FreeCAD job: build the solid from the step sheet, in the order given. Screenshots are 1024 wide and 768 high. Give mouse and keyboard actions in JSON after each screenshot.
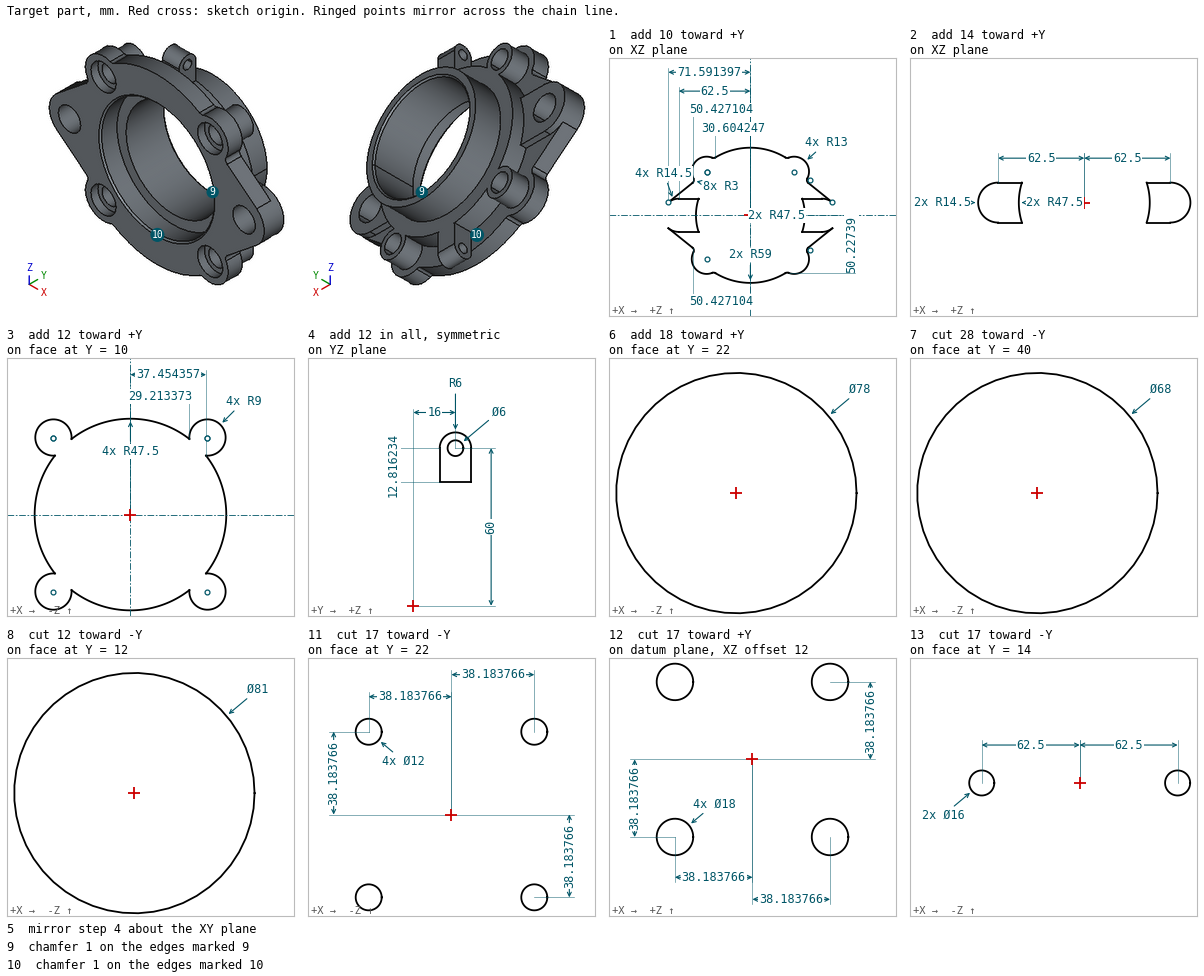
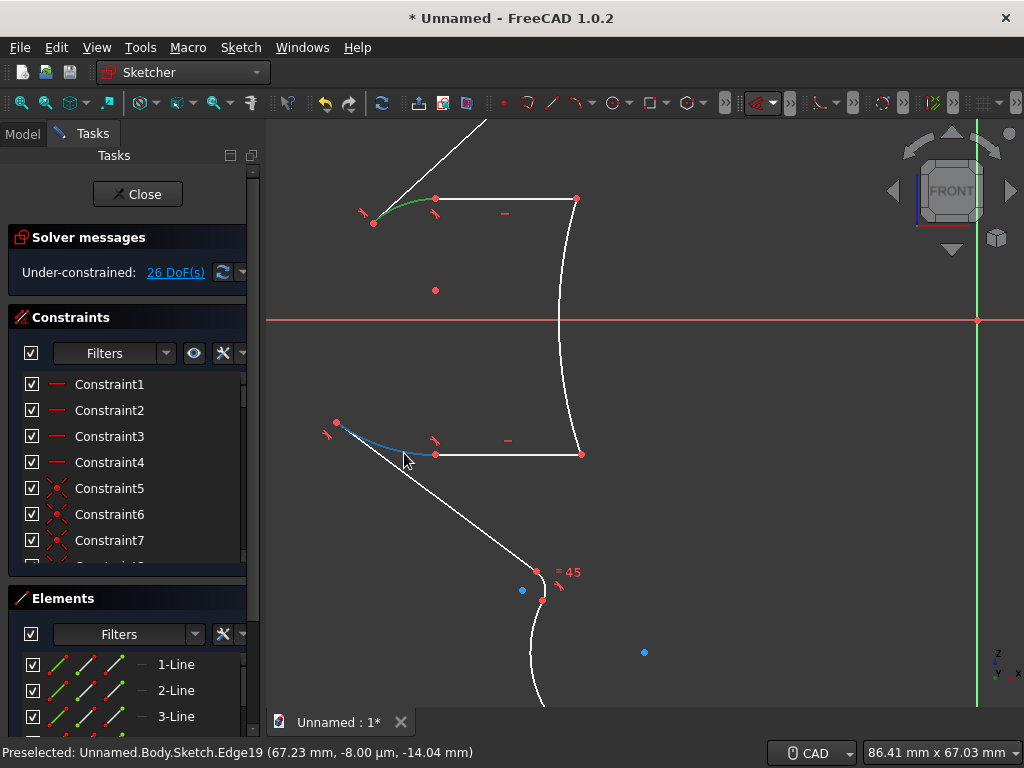
{"action": "left_click", "coordinate": [404, 452]}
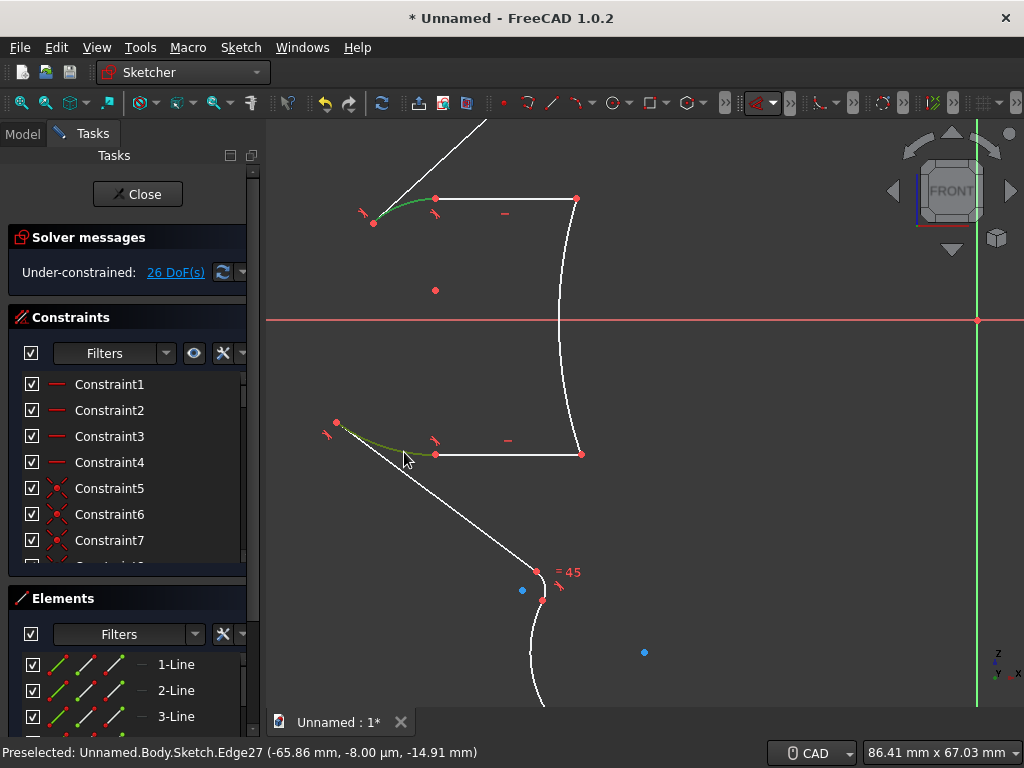
{"action": "key", "text": "e"}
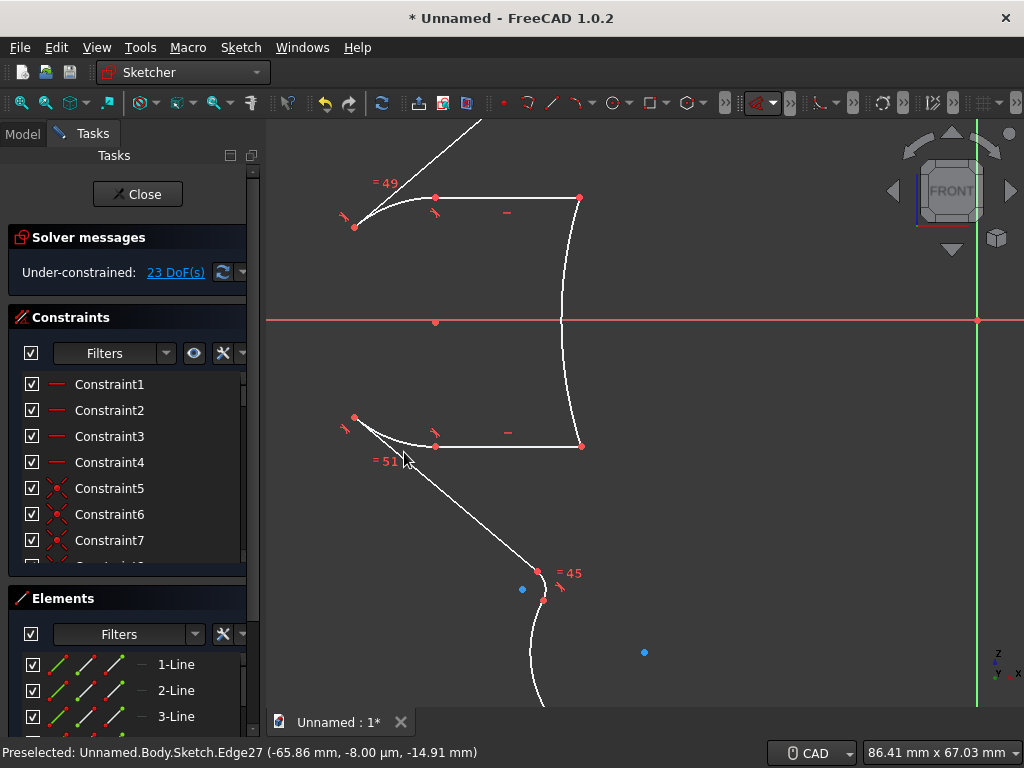
{"action": "scroll", "coordinate": [404, 453], "scroll_direction": "down", "scroll_amount": 6}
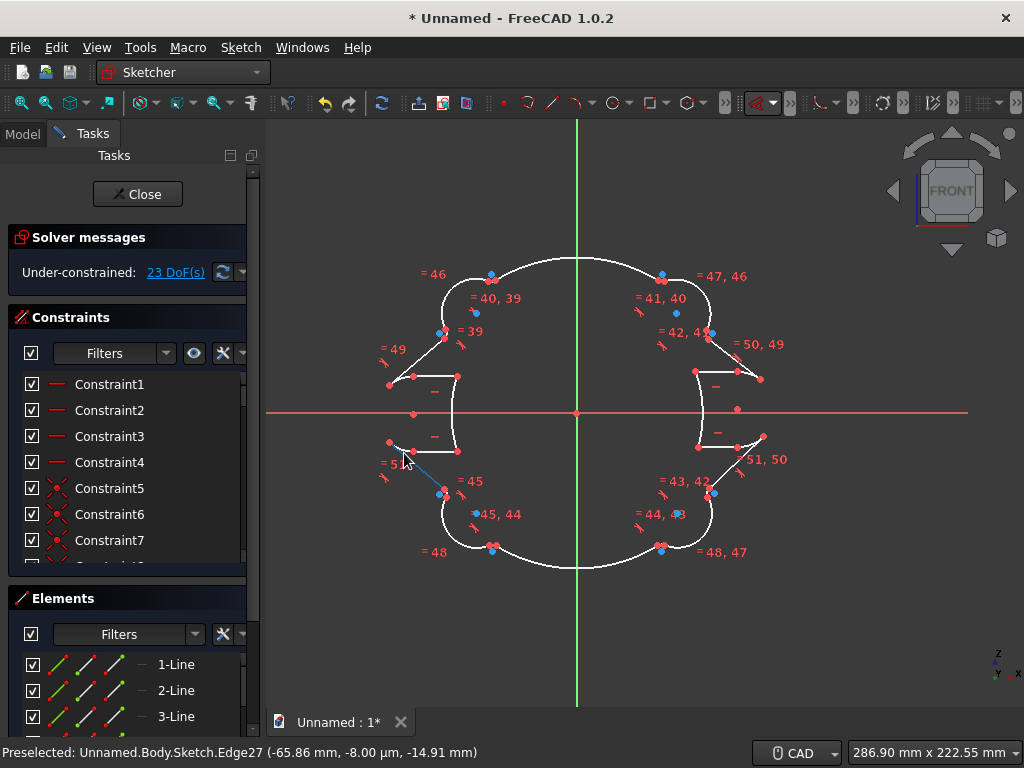
{"action": "left_click", "coordinate": [611, 261]}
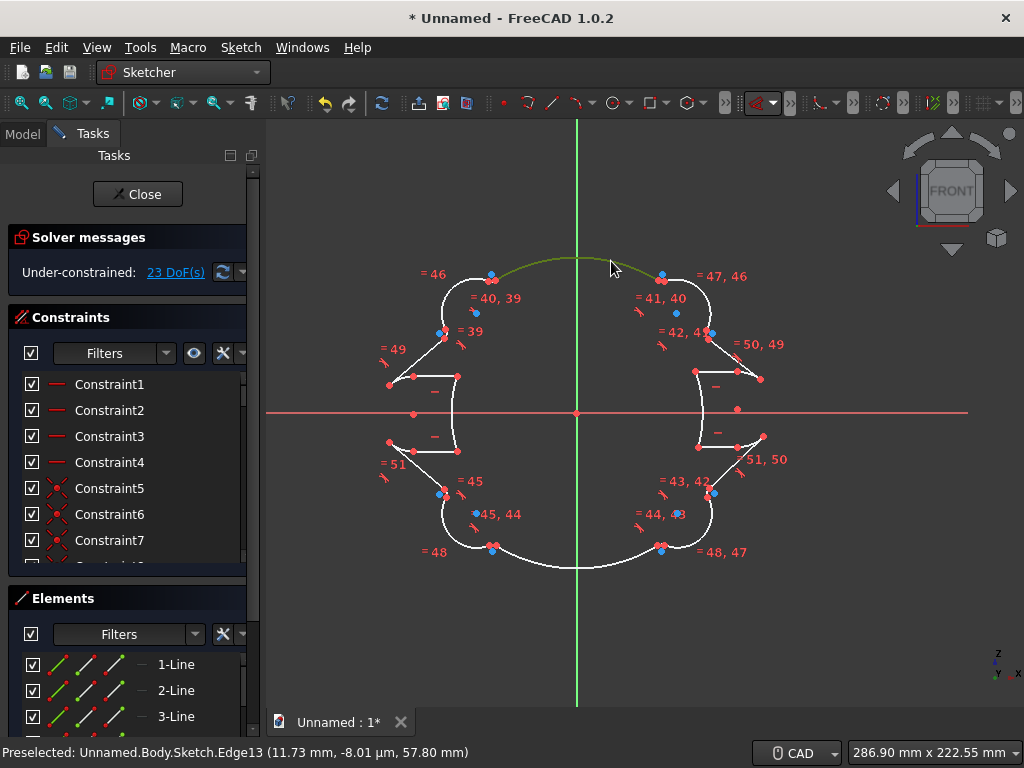
{"action": "left_click", "coordinate": [543, 565]}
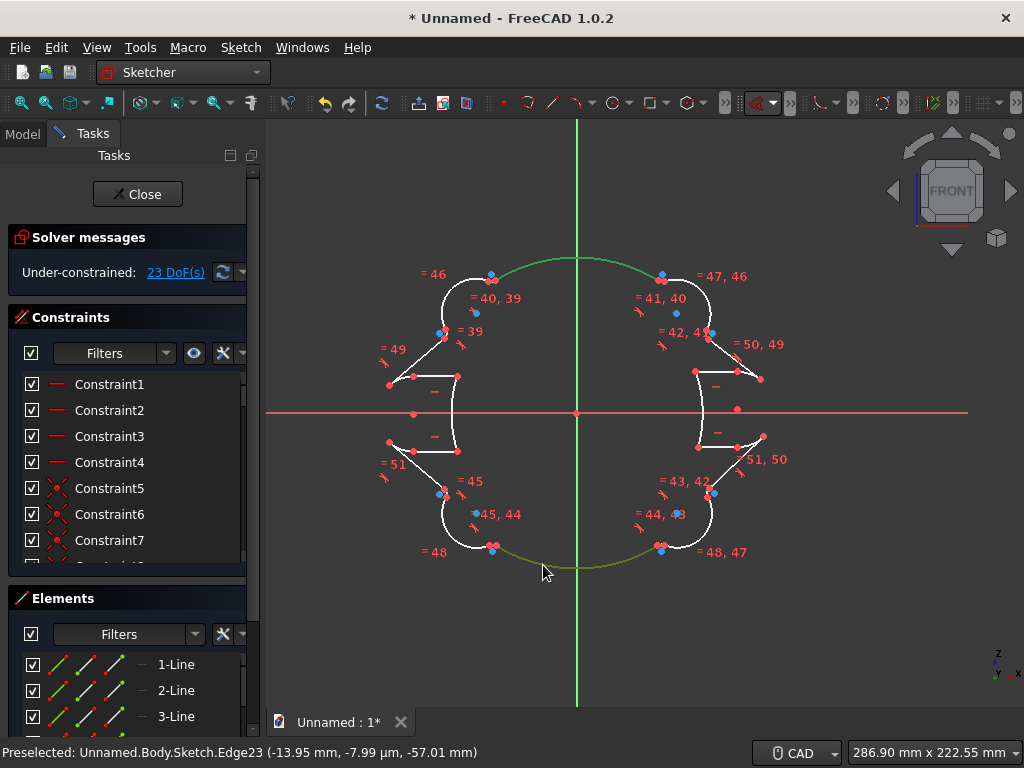
{"action": "key", "text": "e"}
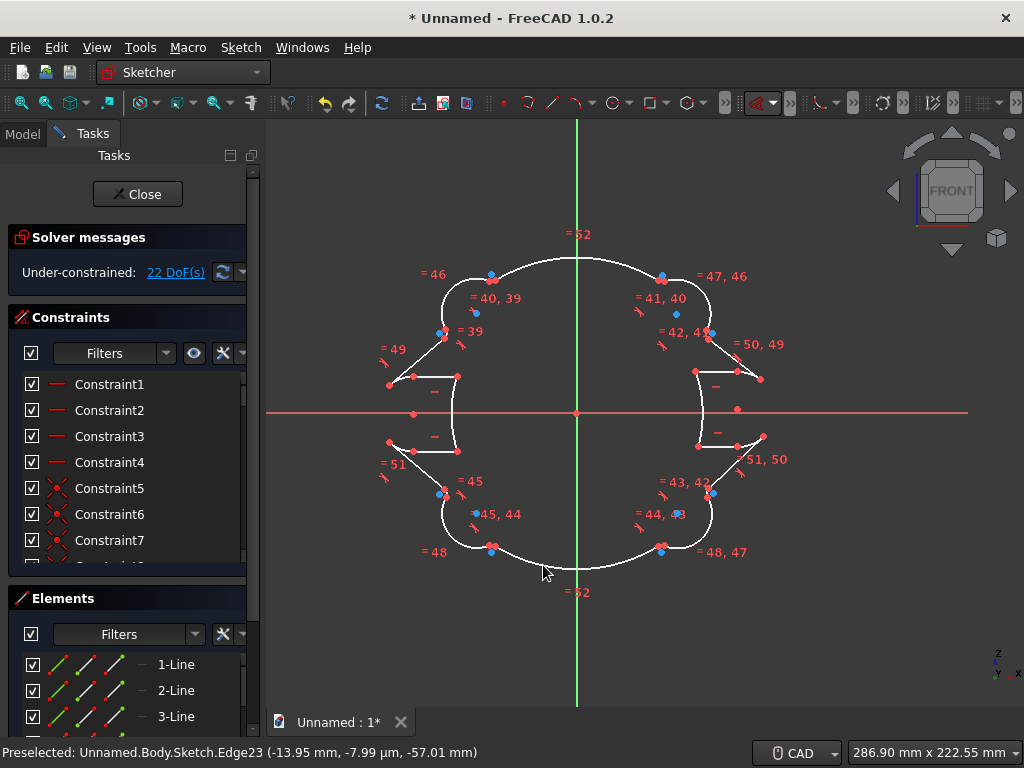
{"action": "scroll", "coordinate": [702, 424], "scroll_direction": "up", "scroll_amount": 2}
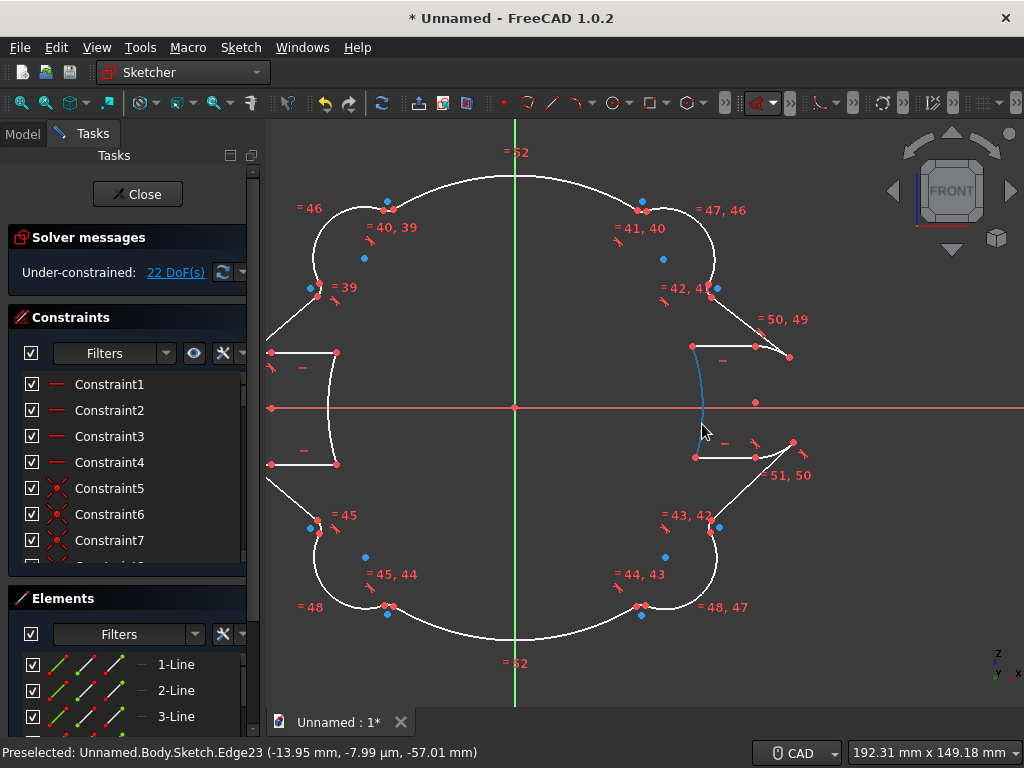
{"action": "left_click", "coordinate": [702, 424]}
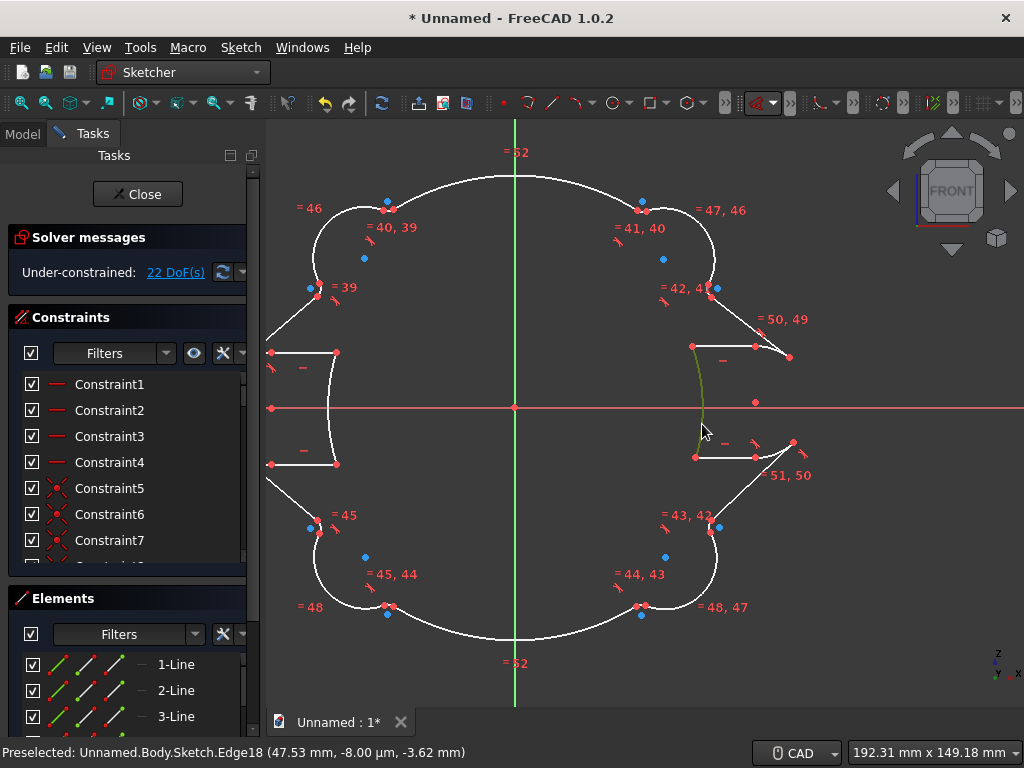
{"action": "left_click", "coordinate": [329, 386]}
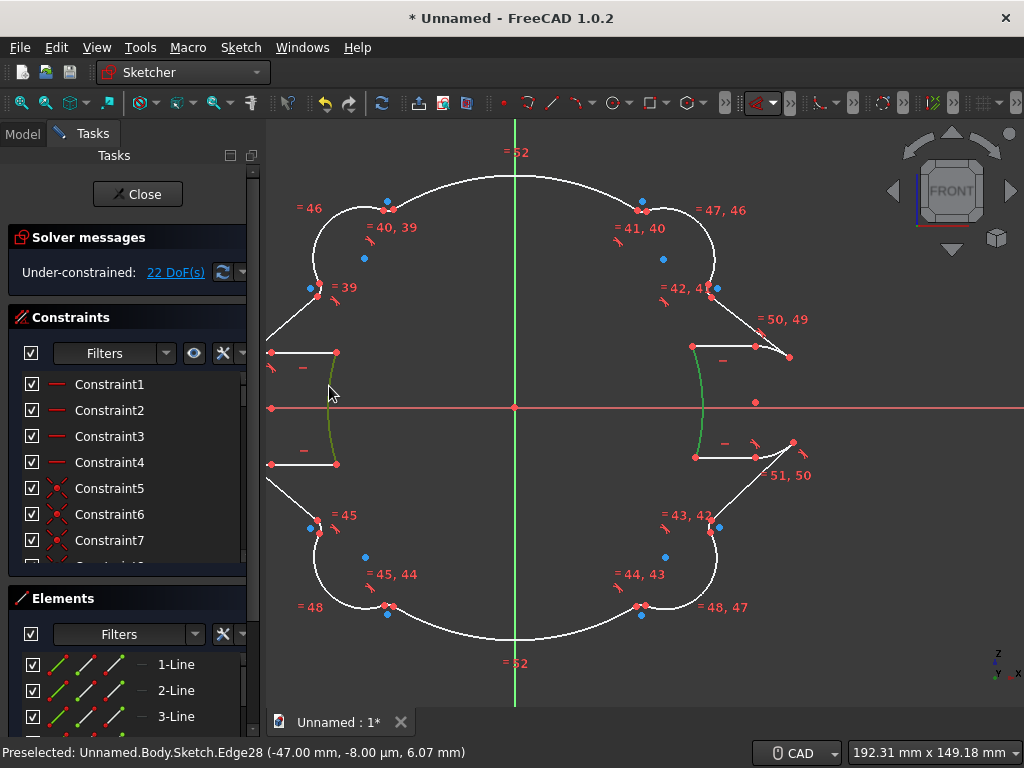
{"action": "key", "text": "e"}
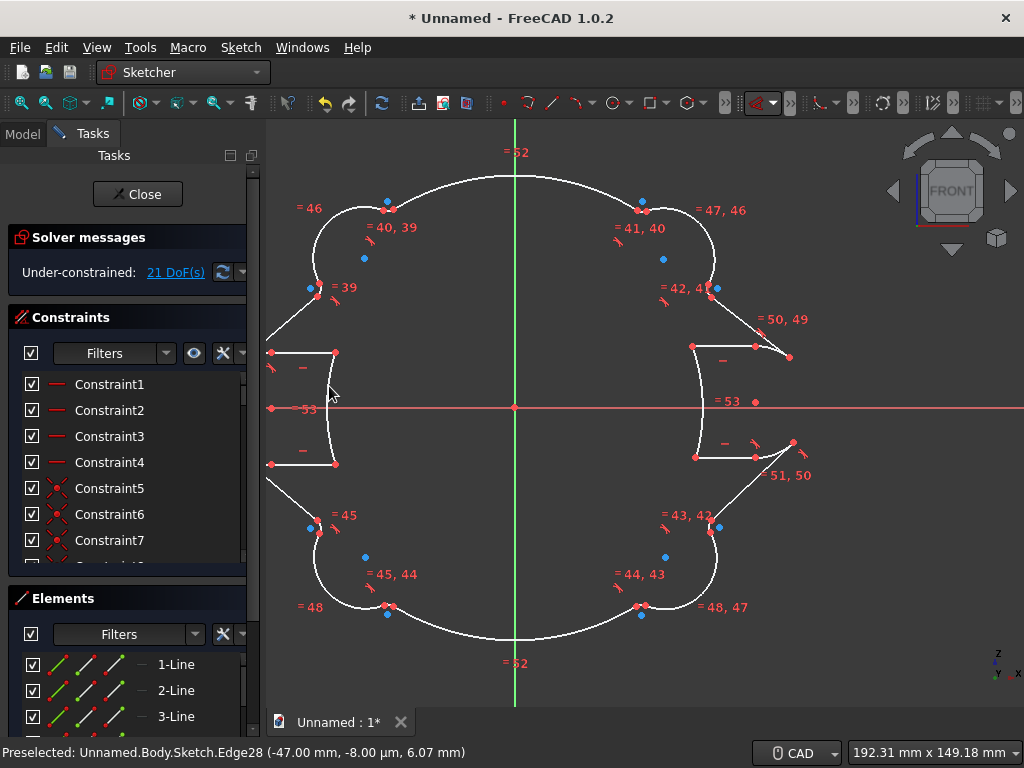
{"action": "scroll", "coordinate": [702, 423], "scroll_direction": "down", "scroll_amount": 2}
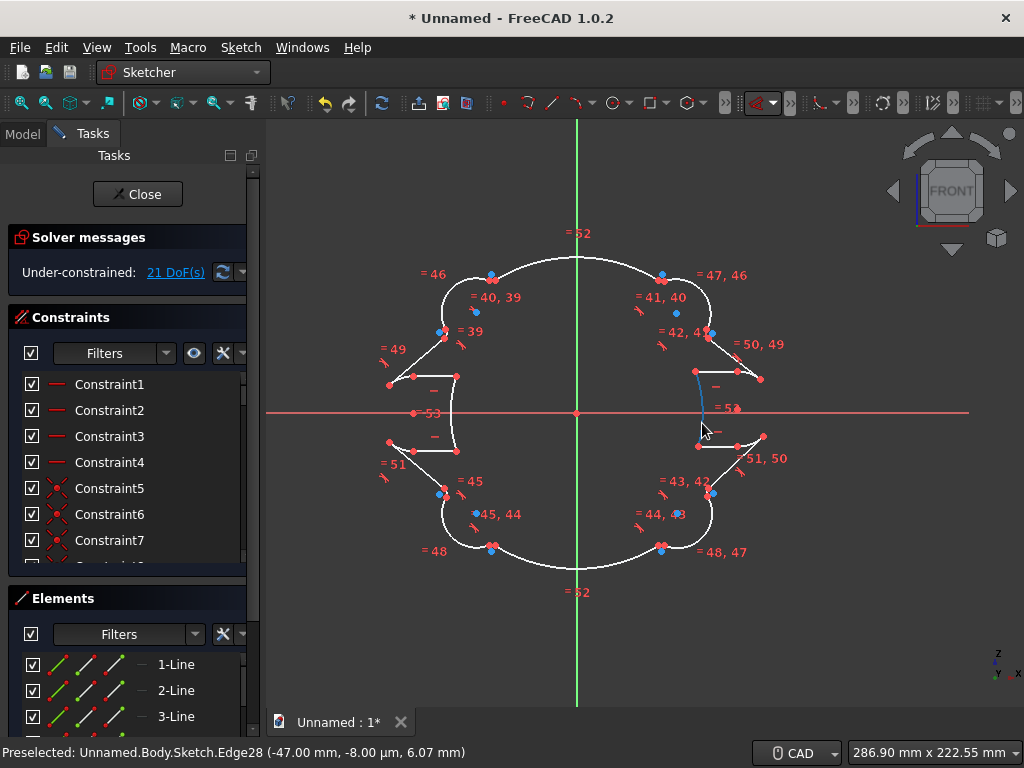
{"action": "left_click", "coordinate": [412, 416]}